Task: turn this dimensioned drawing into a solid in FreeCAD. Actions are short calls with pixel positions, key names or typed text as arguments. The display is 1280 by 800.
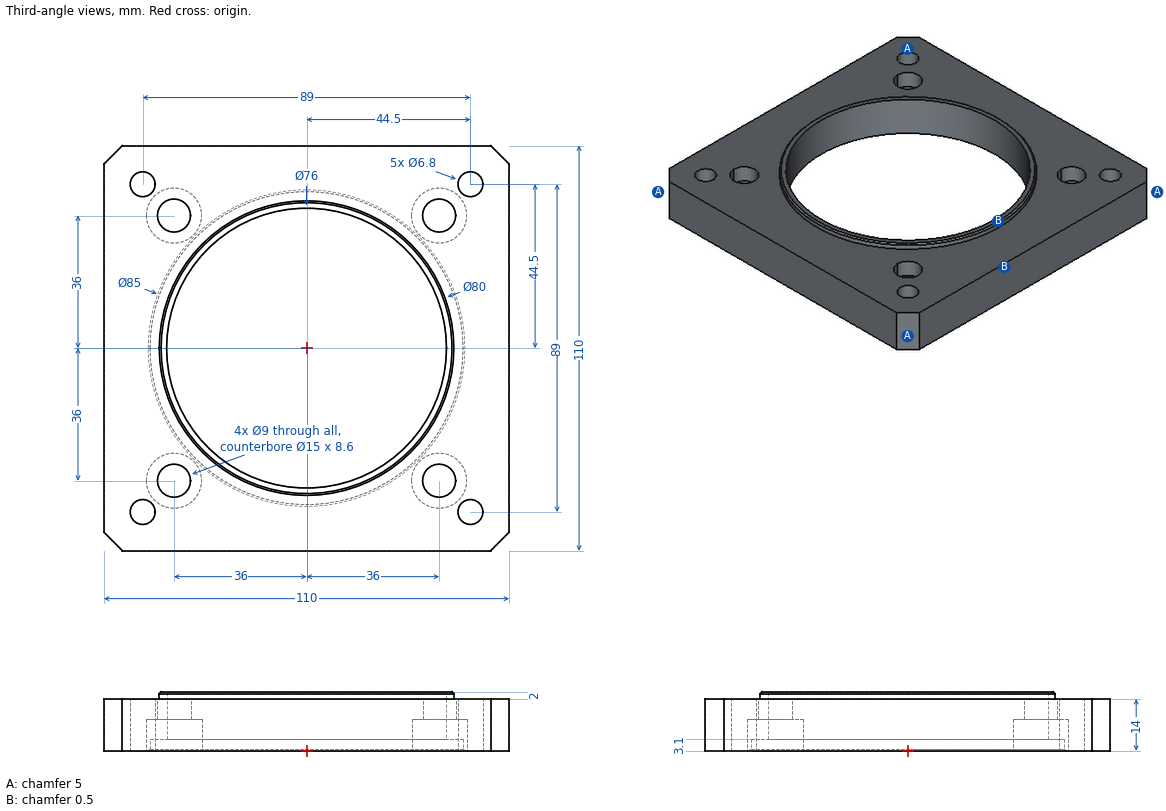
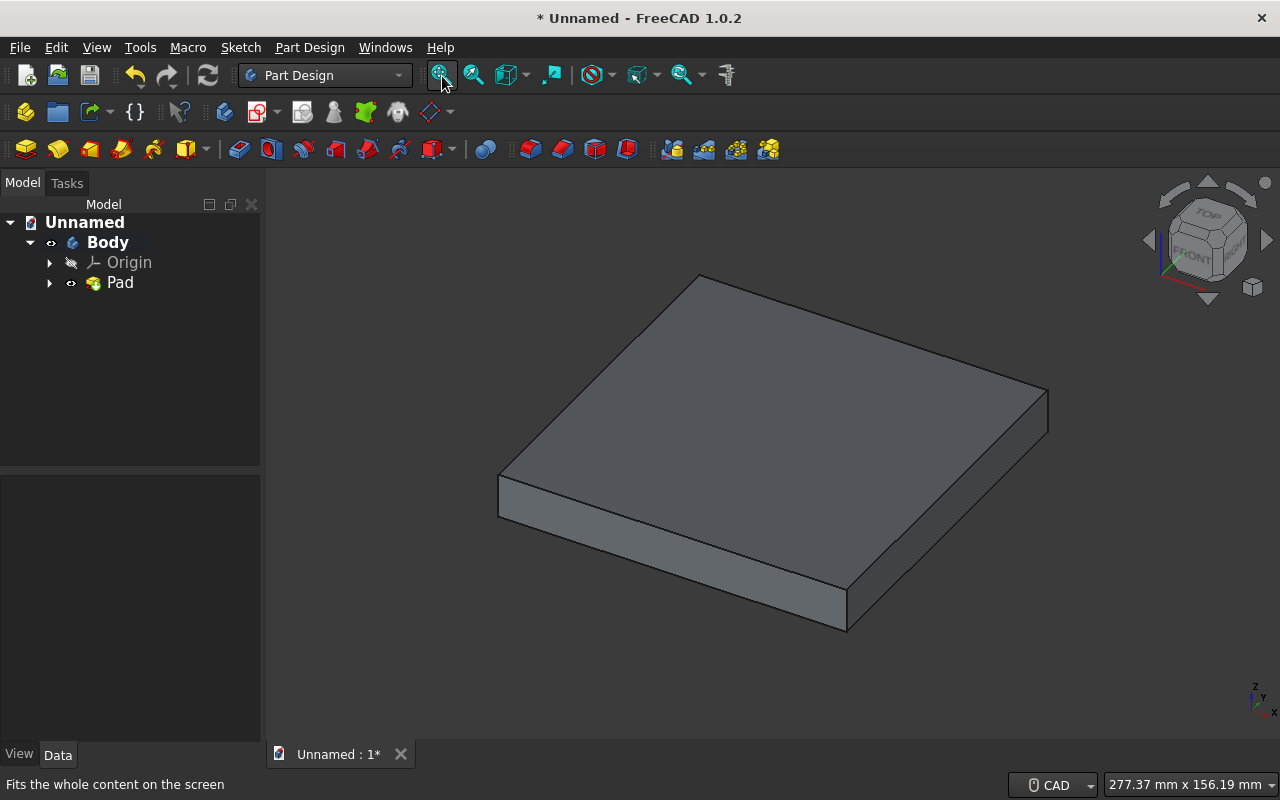
click(773, 432)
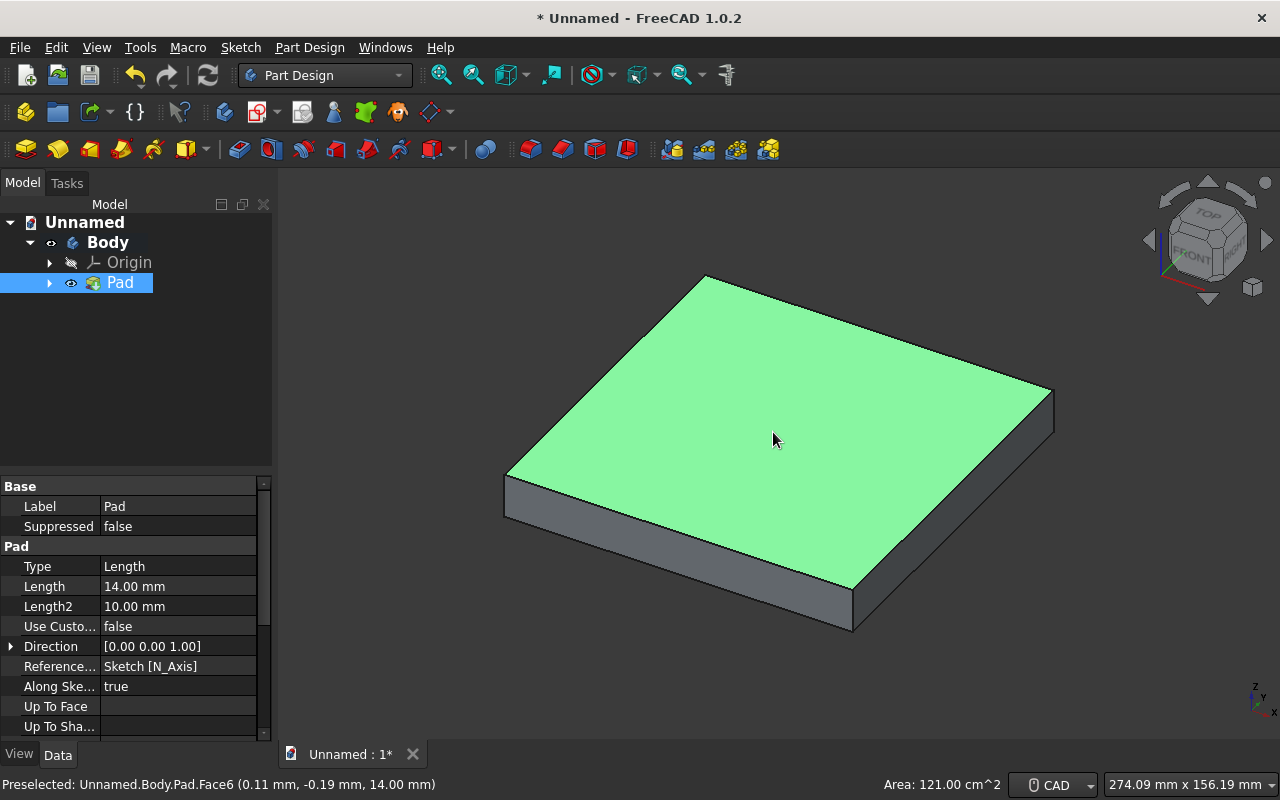
click(258, 112)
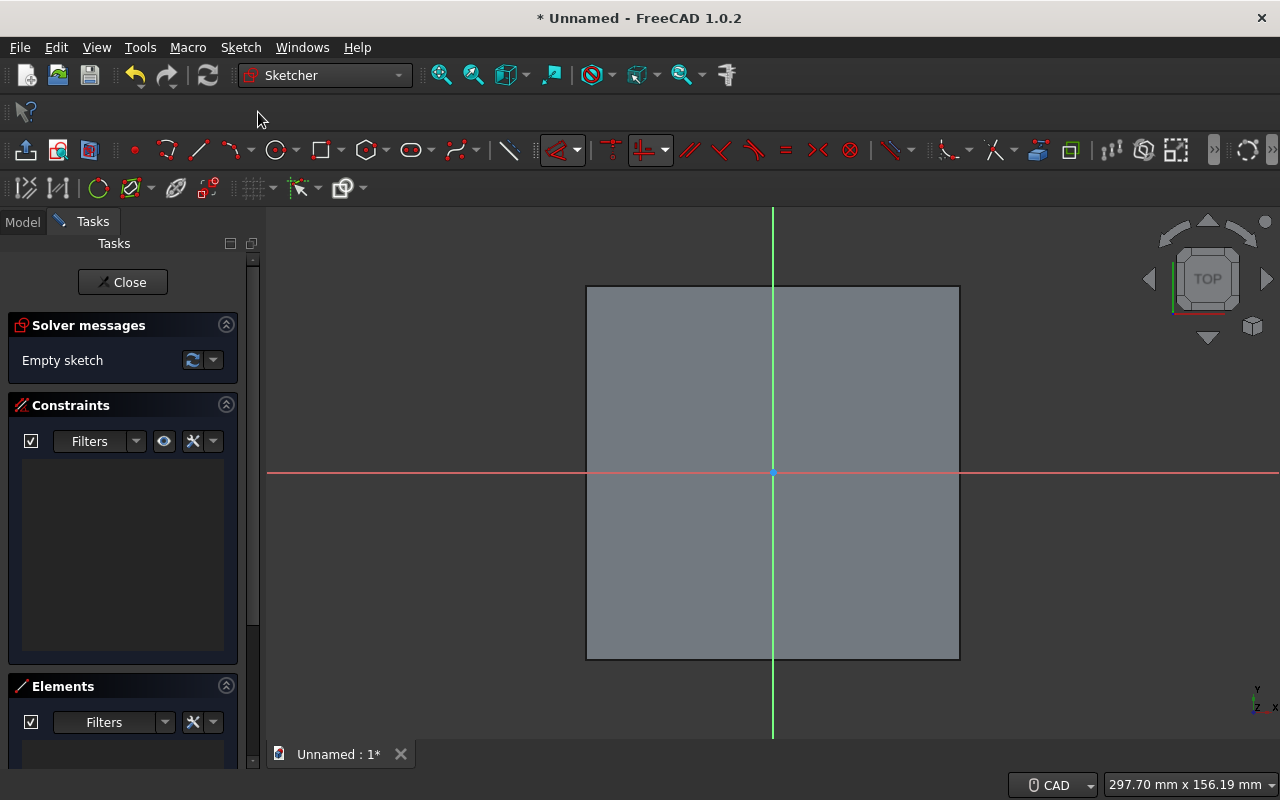
click(276, 150)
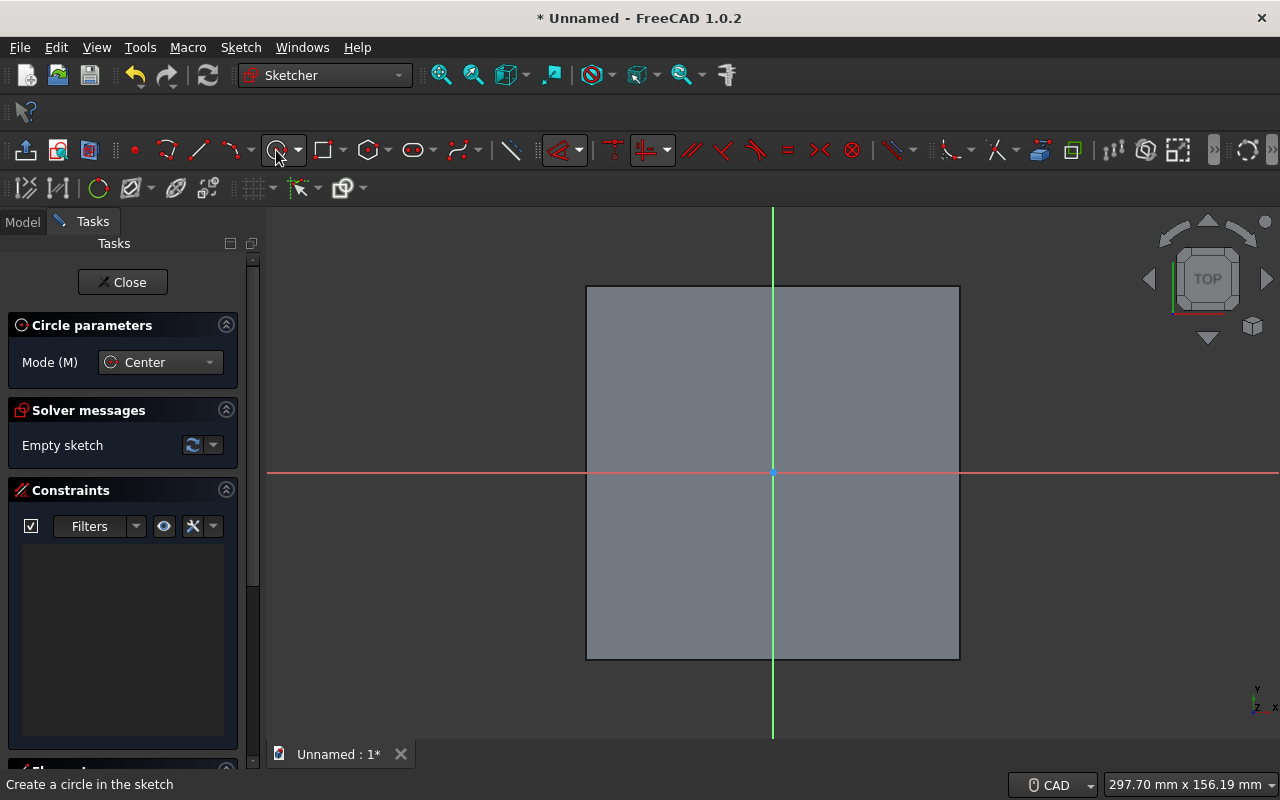
click(773, 473)
click(869, 377)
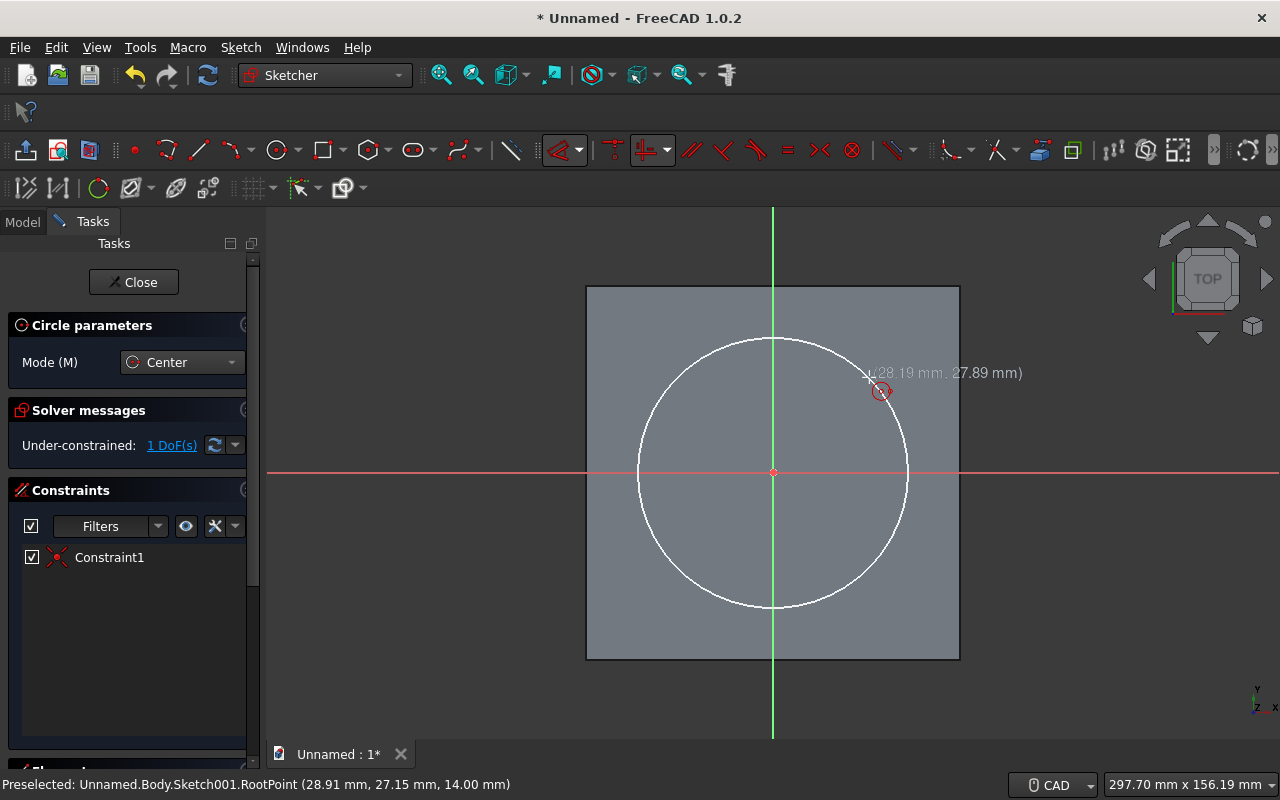
click(773, 473)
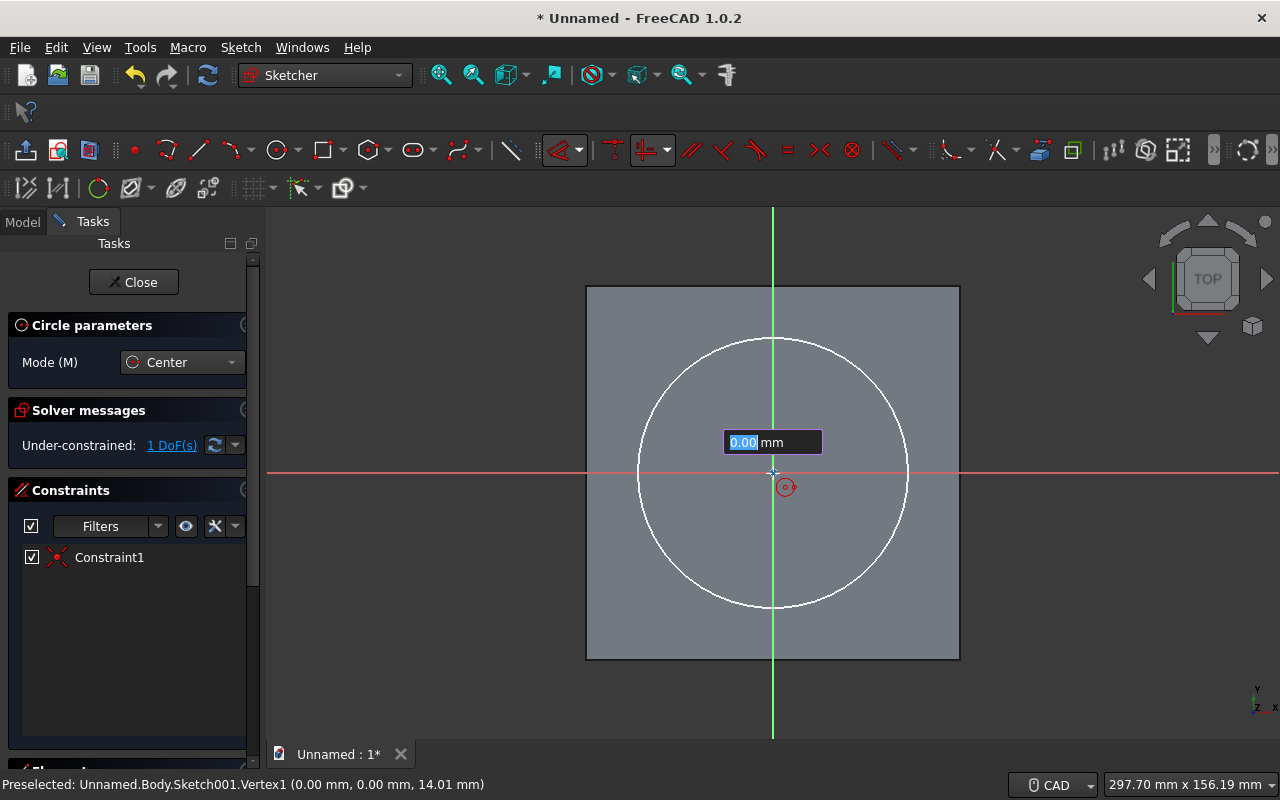
scroll(865, 381, up, 5)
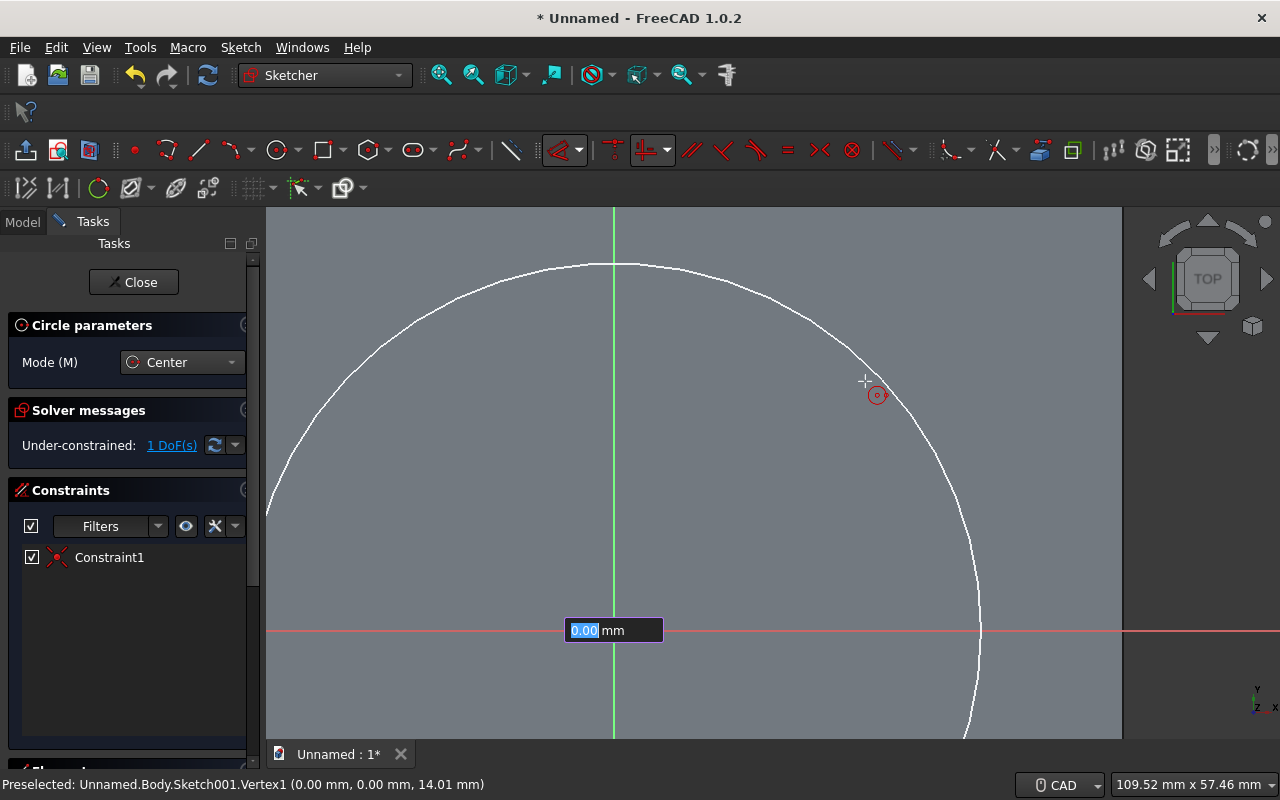
click(863, 382)
key(Escape)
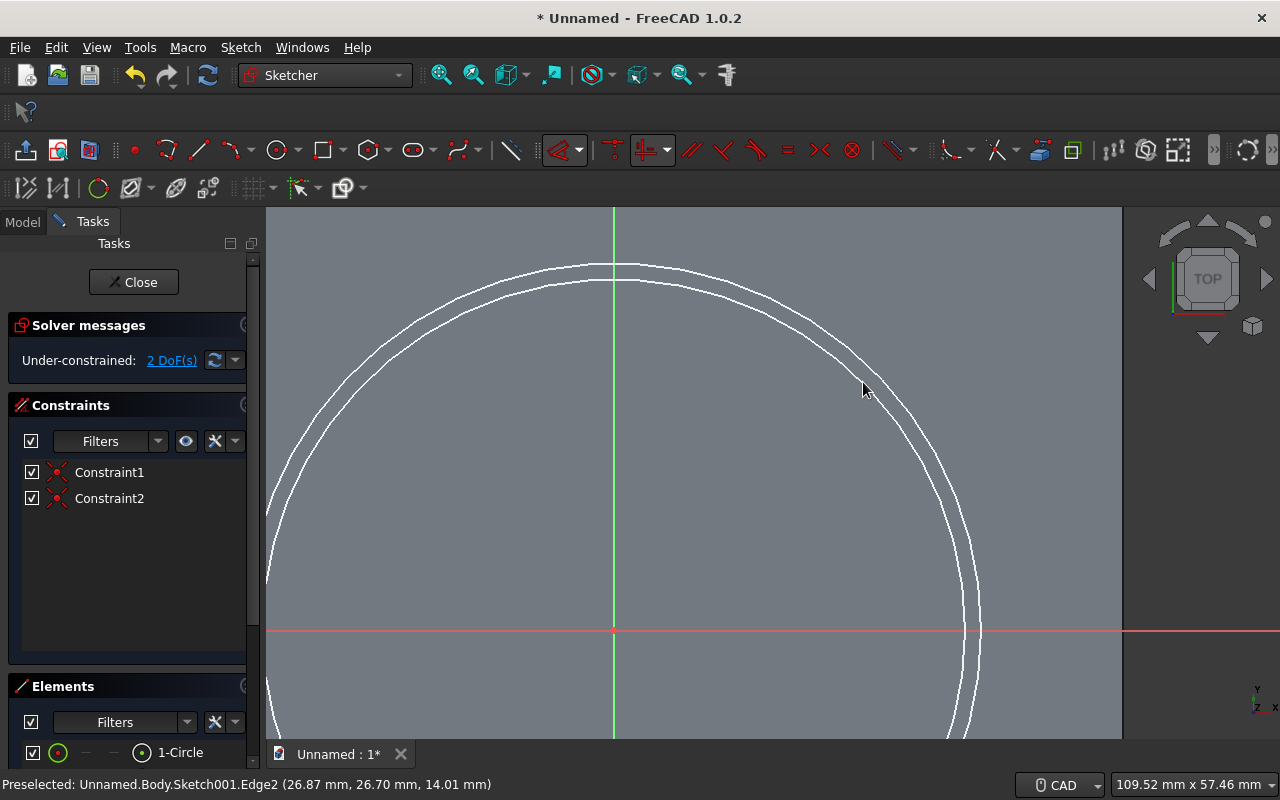
click(873, 370)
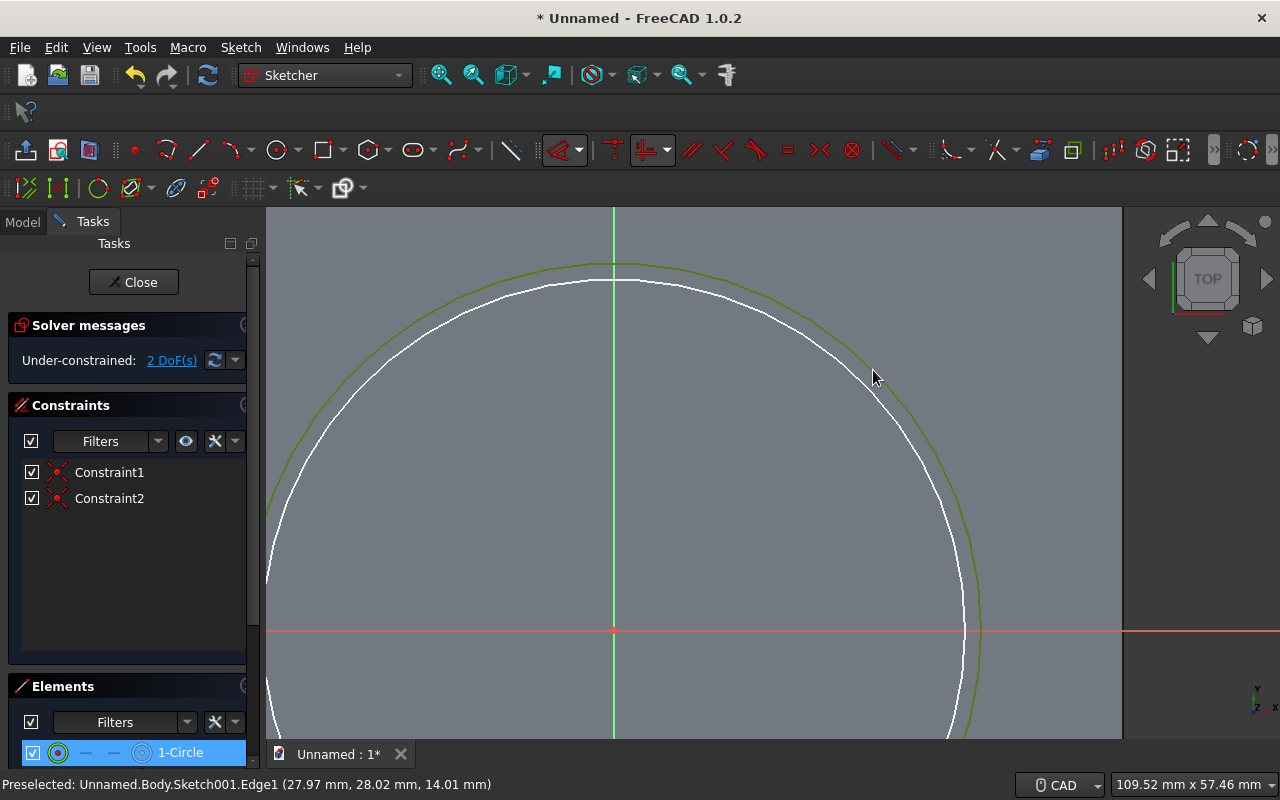
key(k)
key(o)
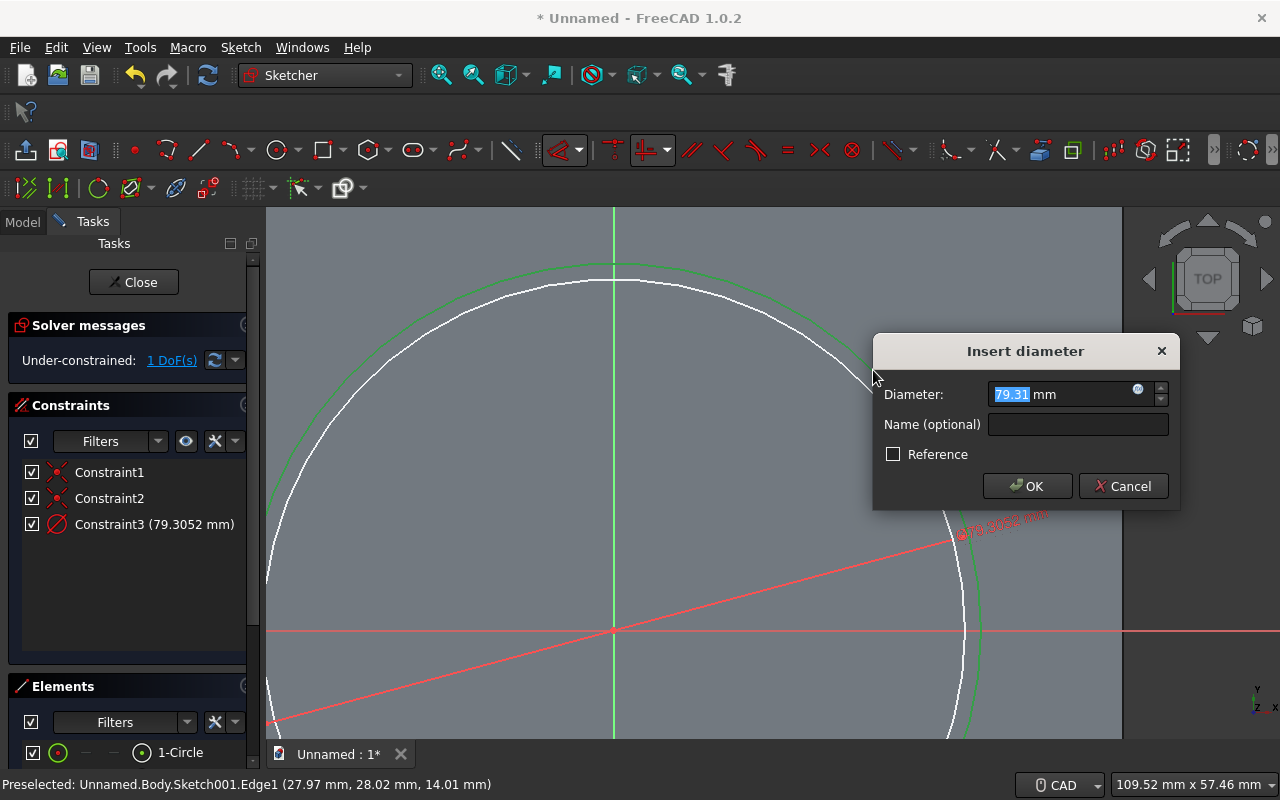
text(80)
key(Return)